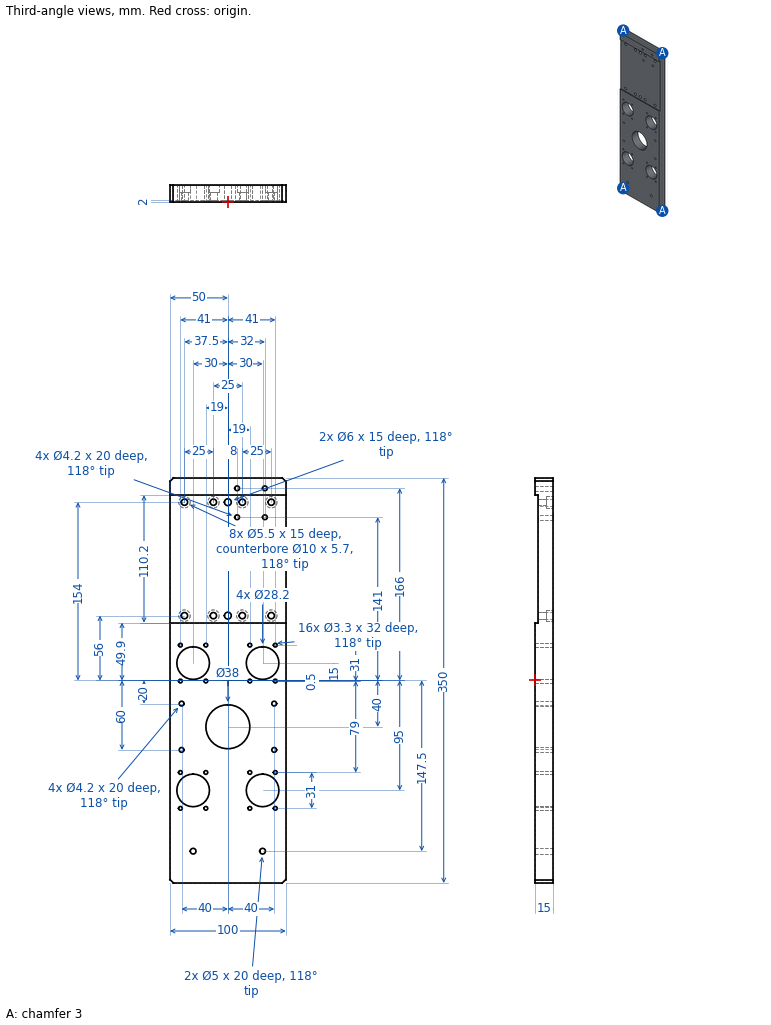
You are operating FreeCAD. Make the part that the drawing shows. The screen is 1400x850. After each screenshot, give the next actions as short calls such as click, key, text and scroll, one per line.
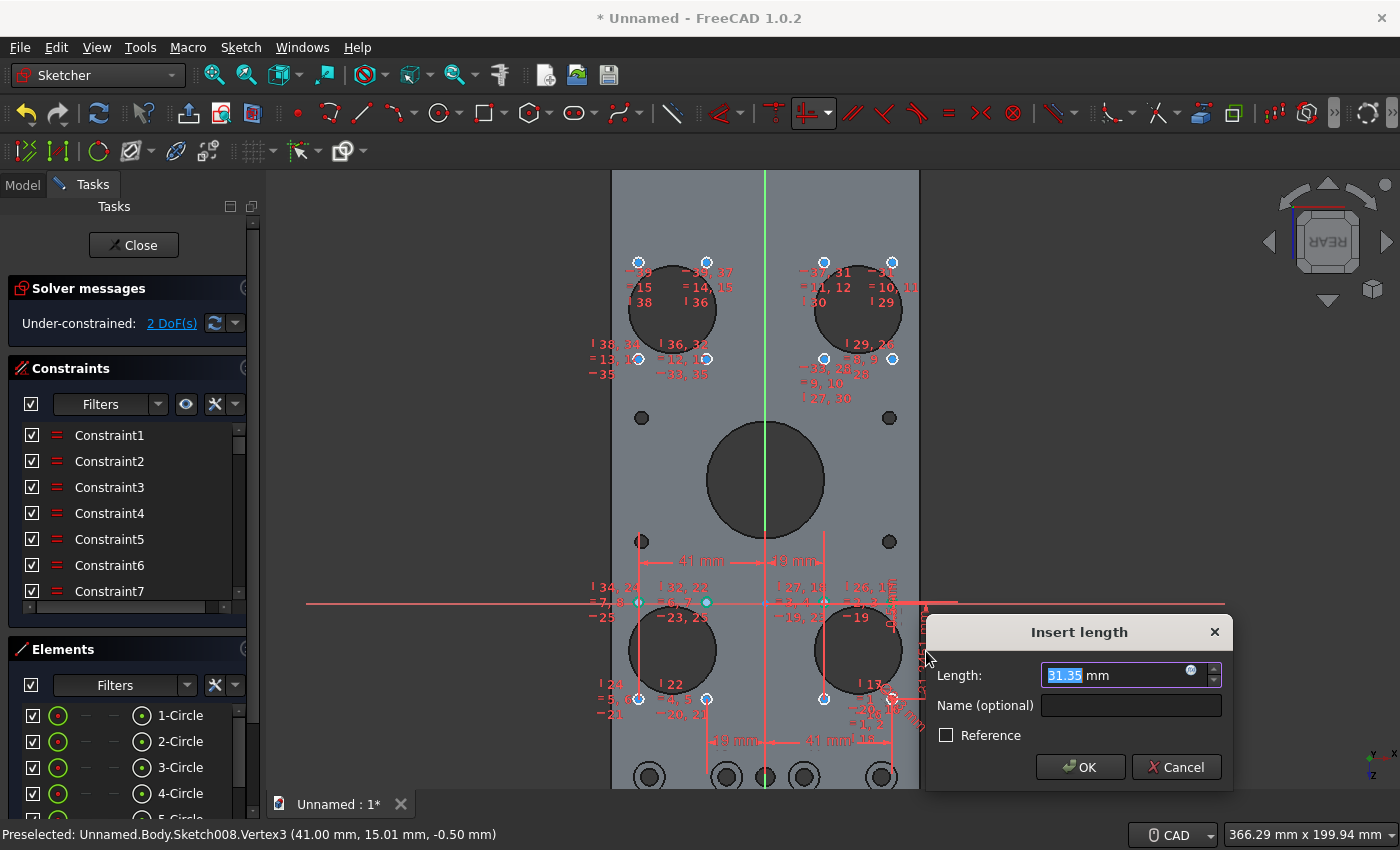
text(31)
key(Return)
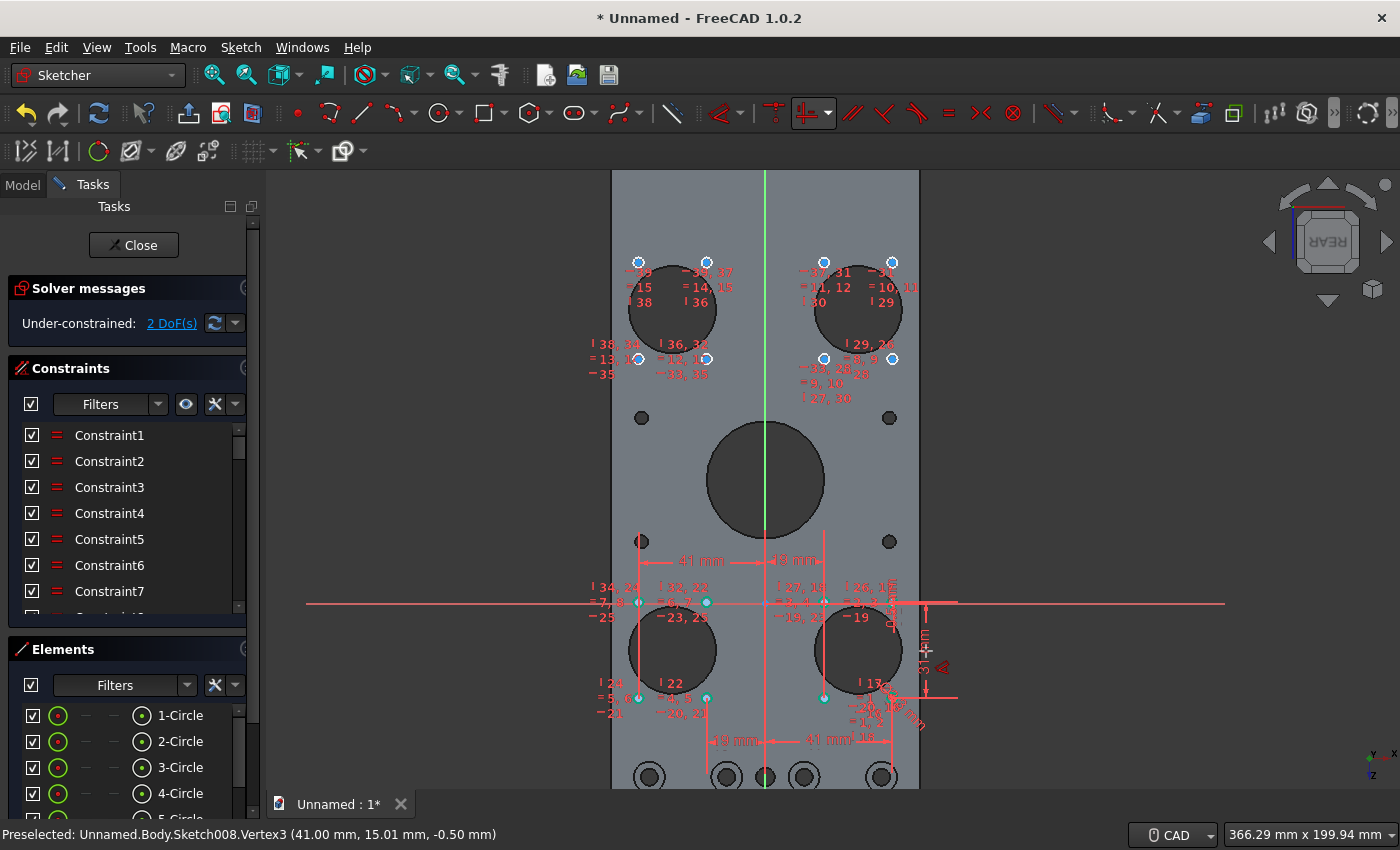
click(892, 602)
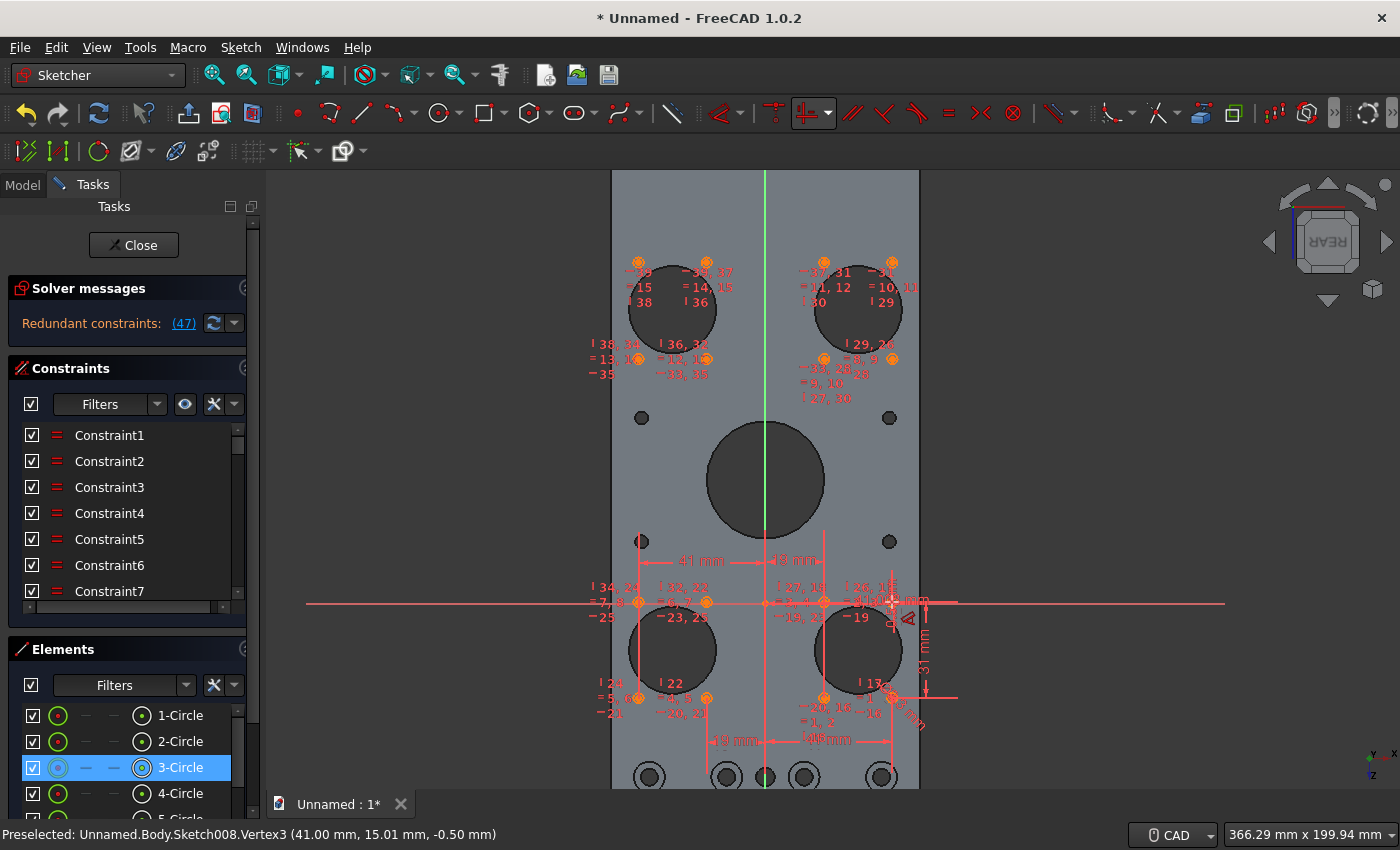
click(892, 359)
click(926, 481)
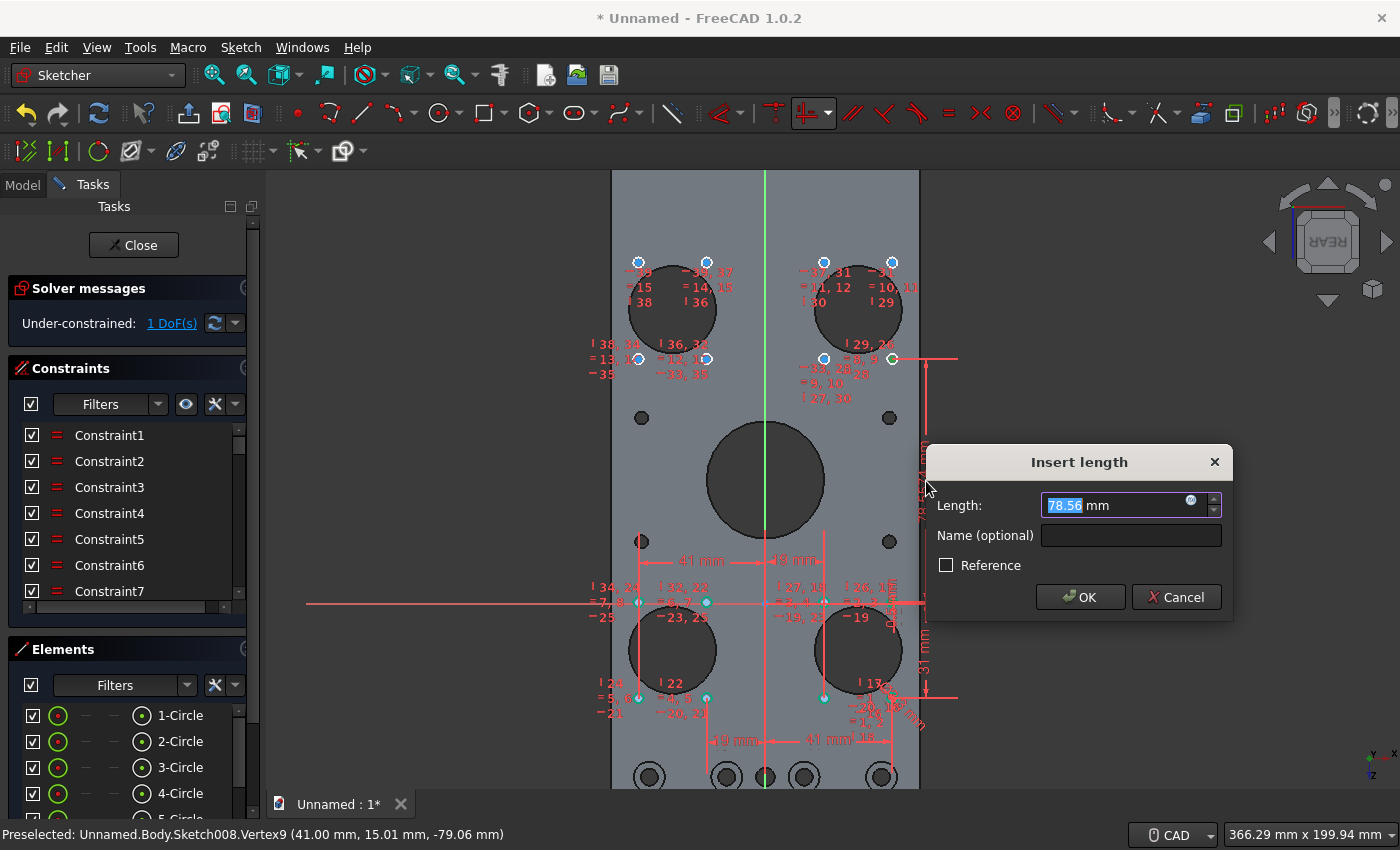
text(79)
key(Return)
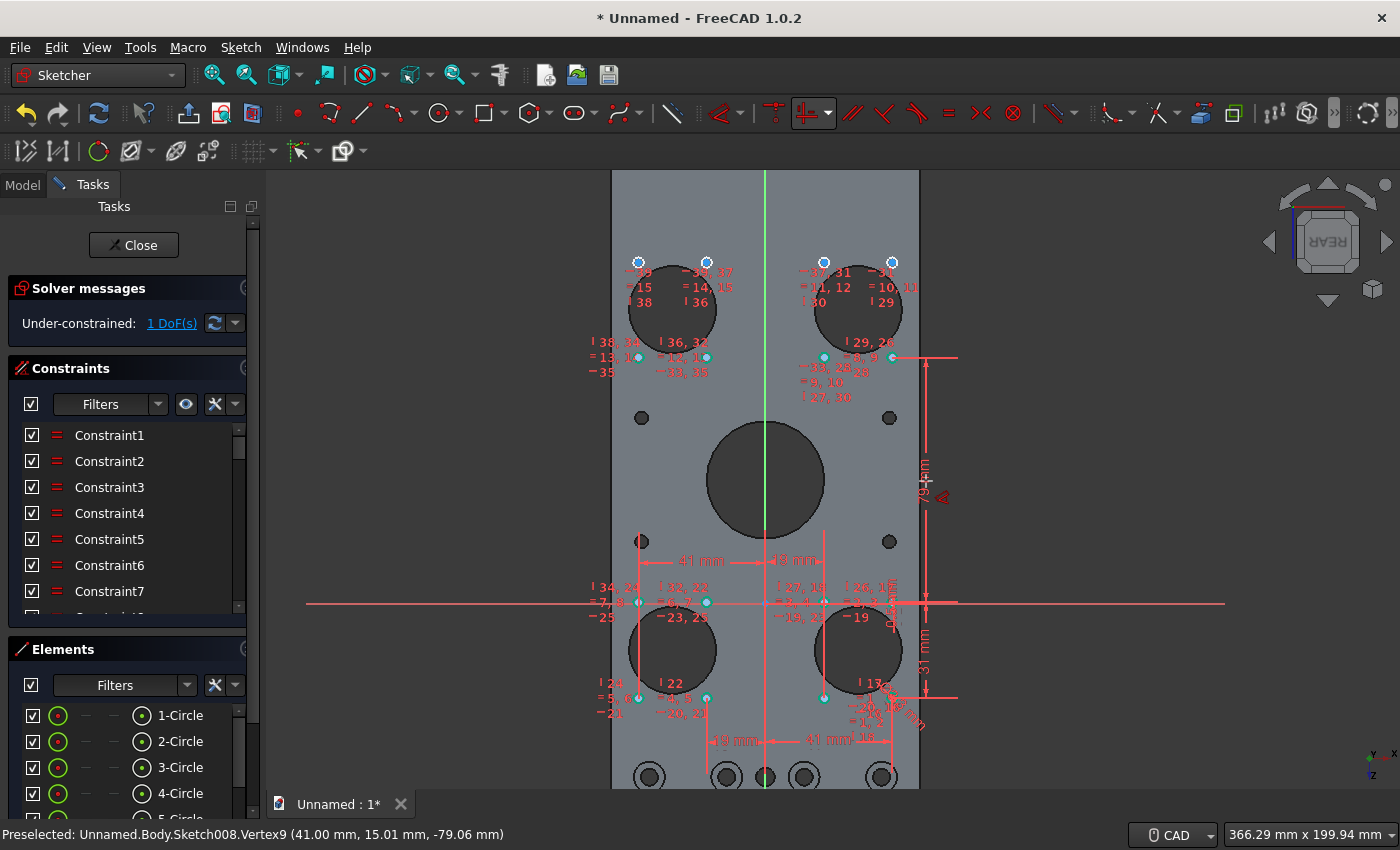
click(892, 358)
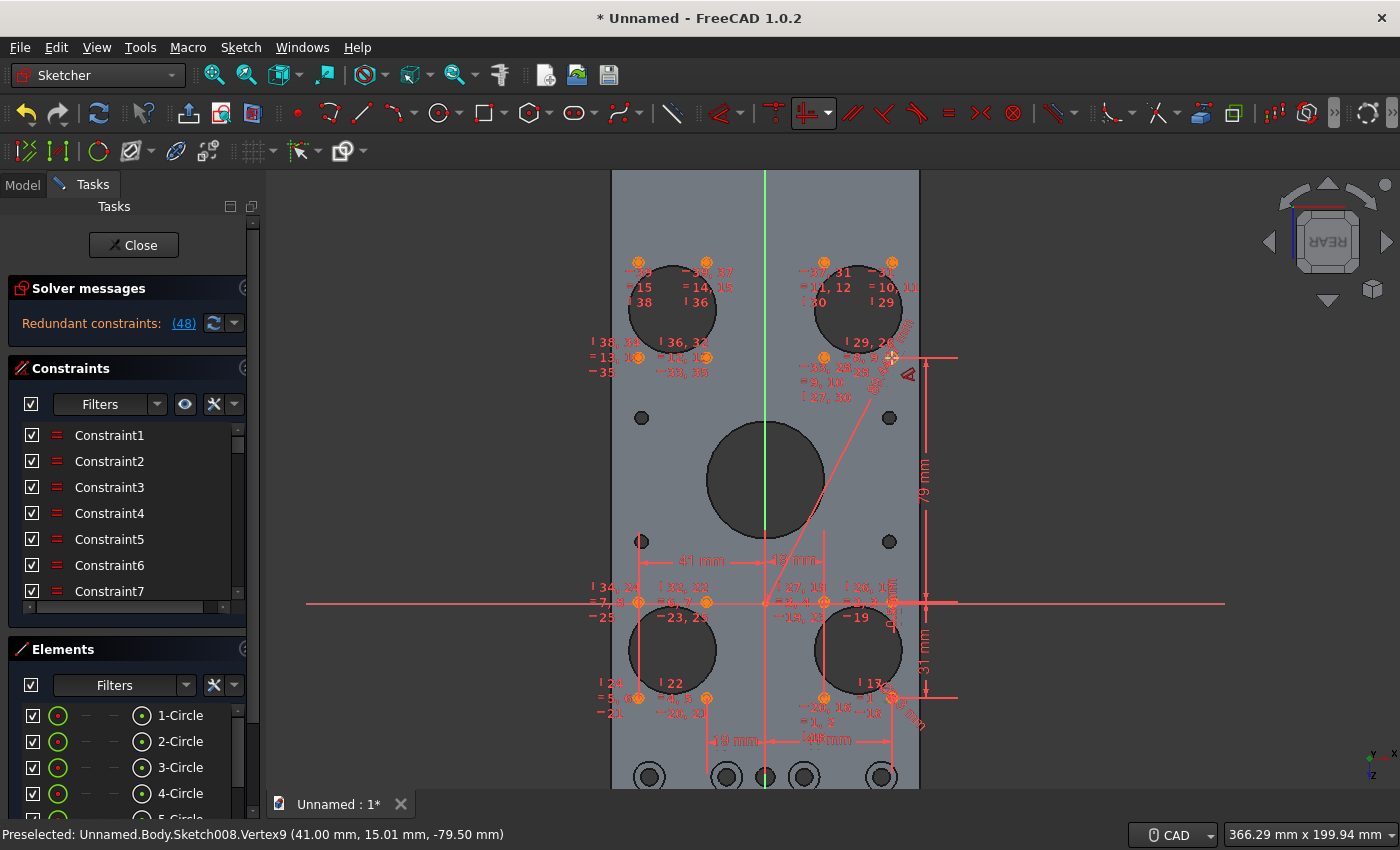
click(892, 263)
click(926, 310)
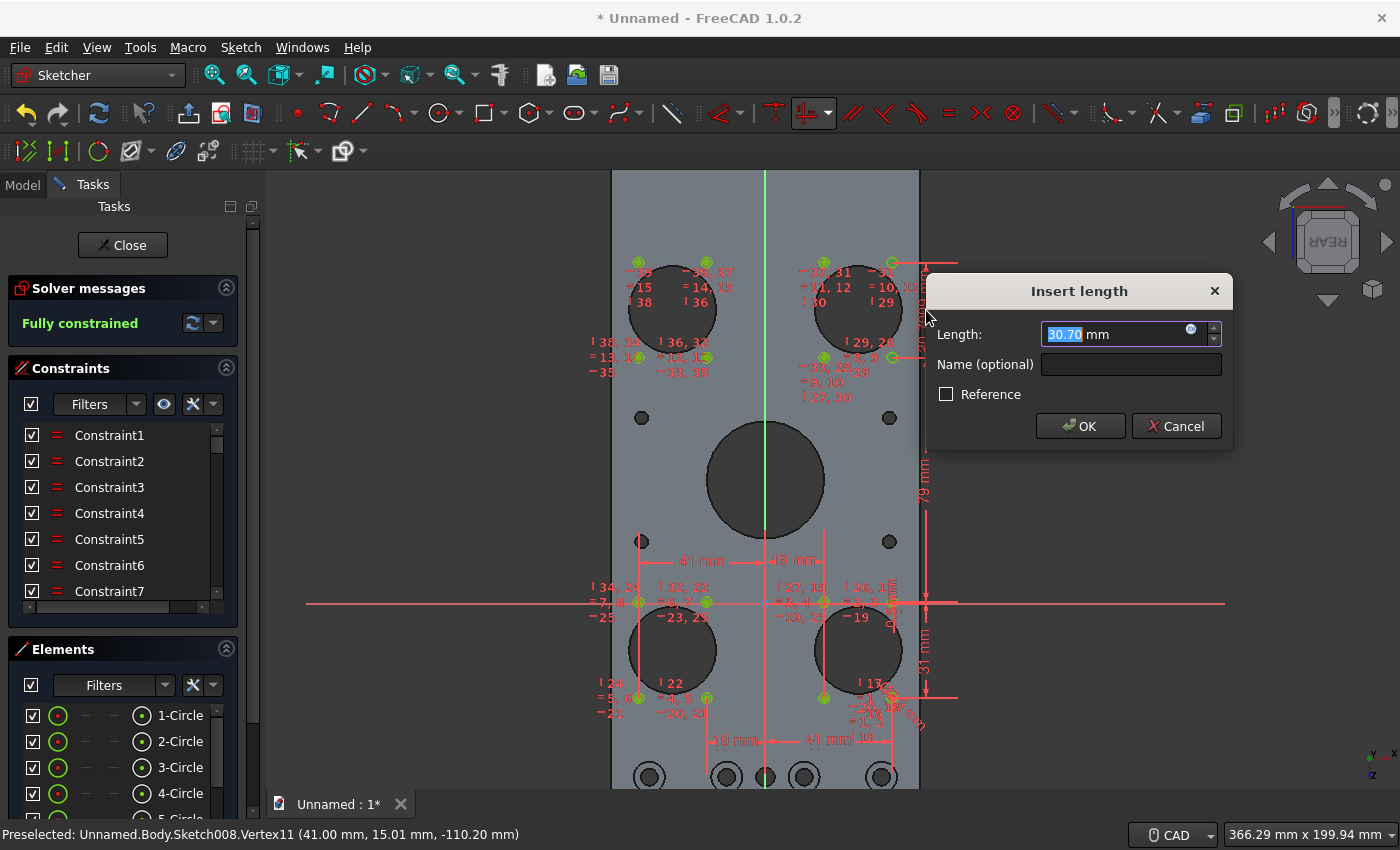
text(31)
key(Return)
key(Escape)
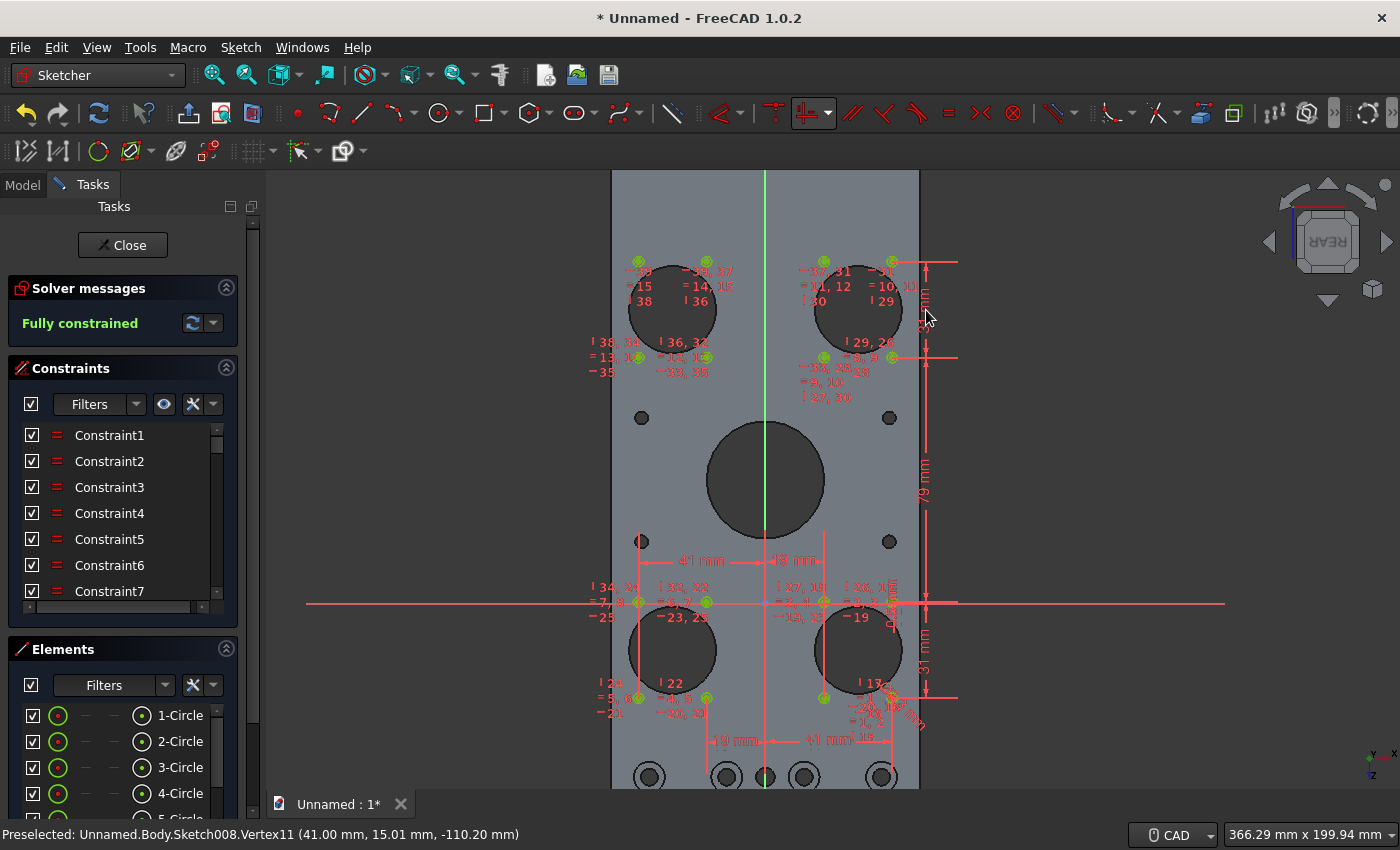
click(123, 245)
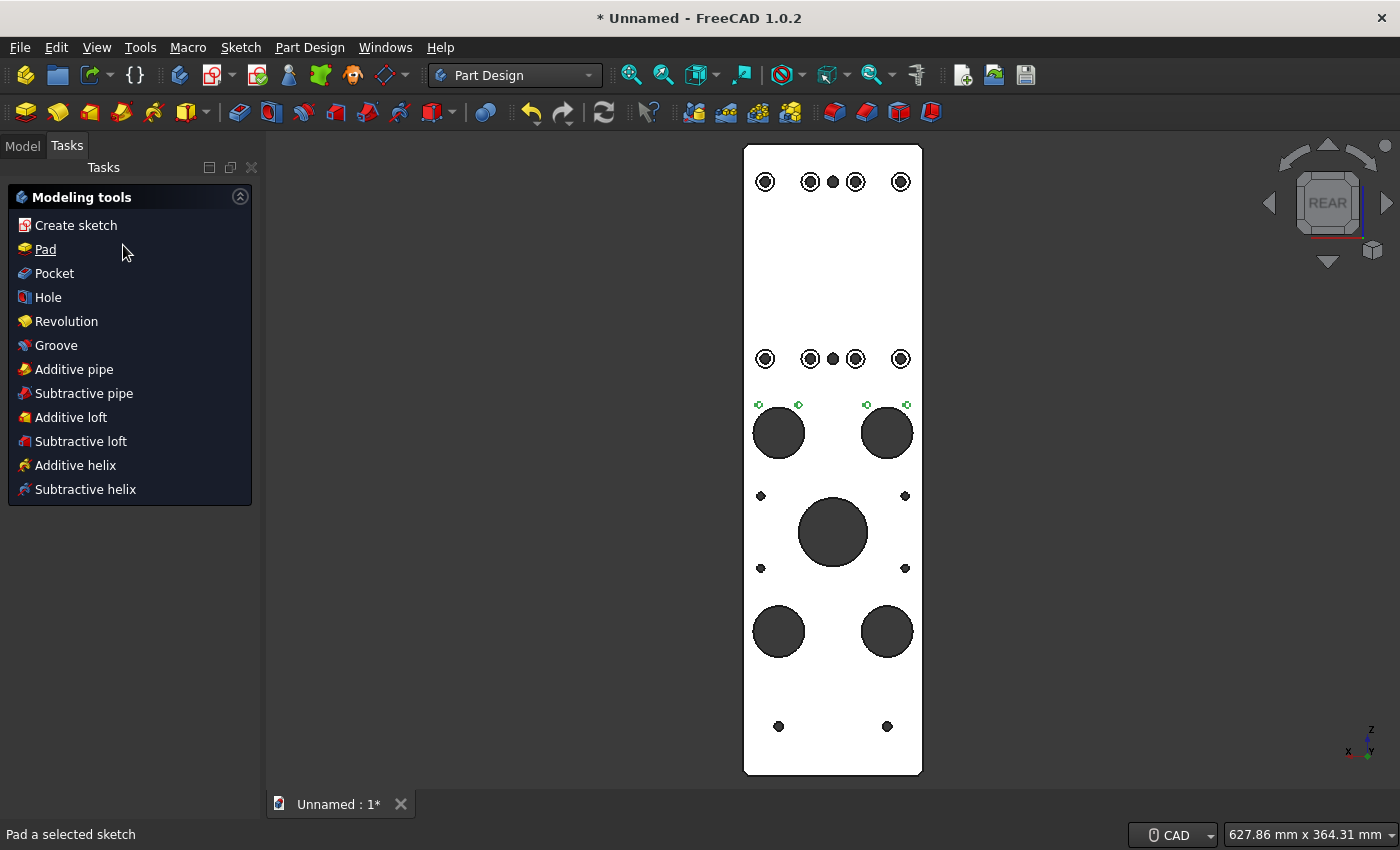
click(272, 112)